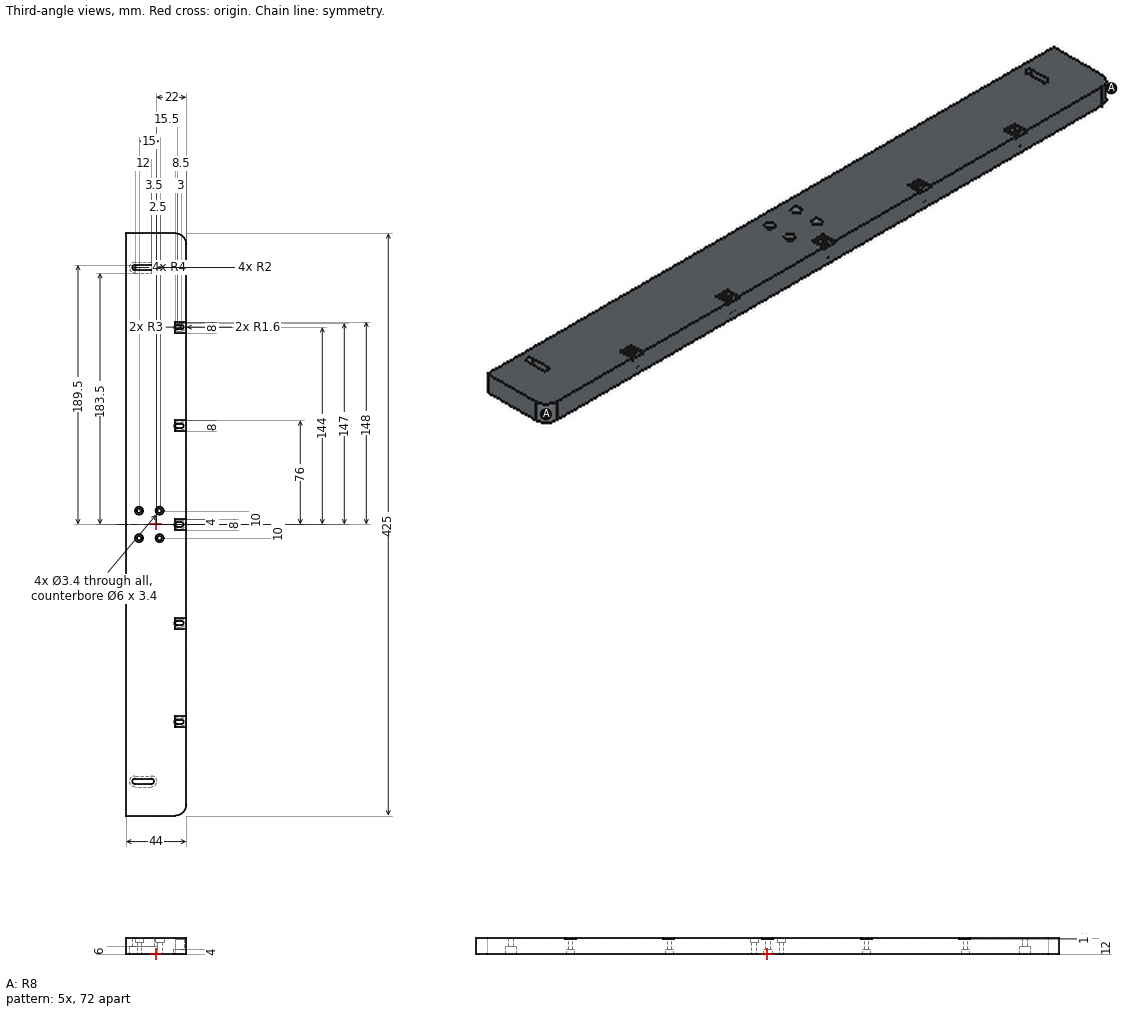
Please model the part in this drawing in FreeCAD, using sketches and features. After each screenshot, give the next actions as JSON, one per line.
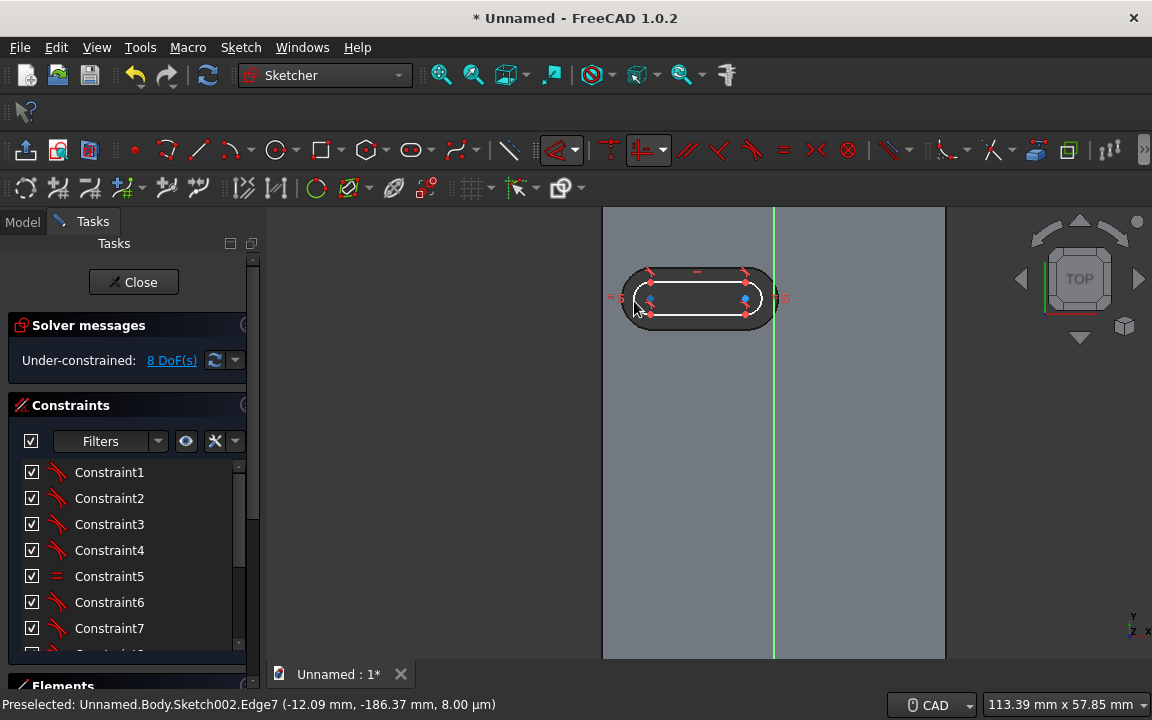
{"action": "left_click", "coordinate": [634, 299]}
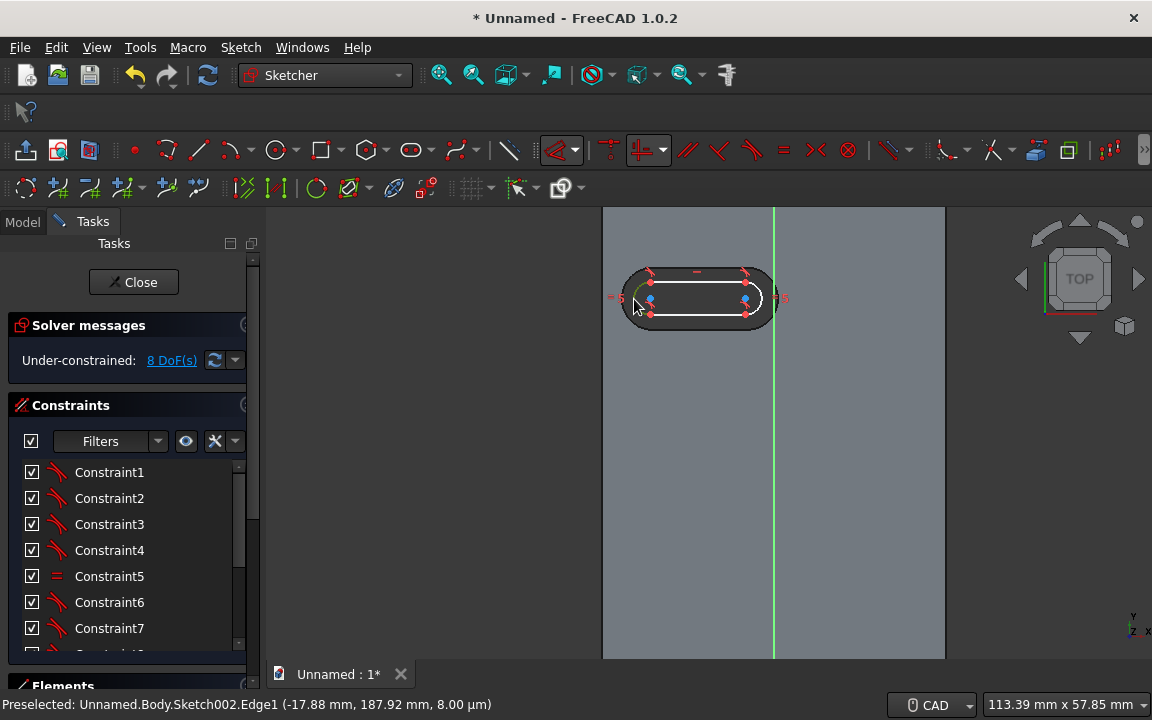
{"action": "scroll", "coordinate": [634, 300], "scroll_direction": "down", "scroll_amount": 12}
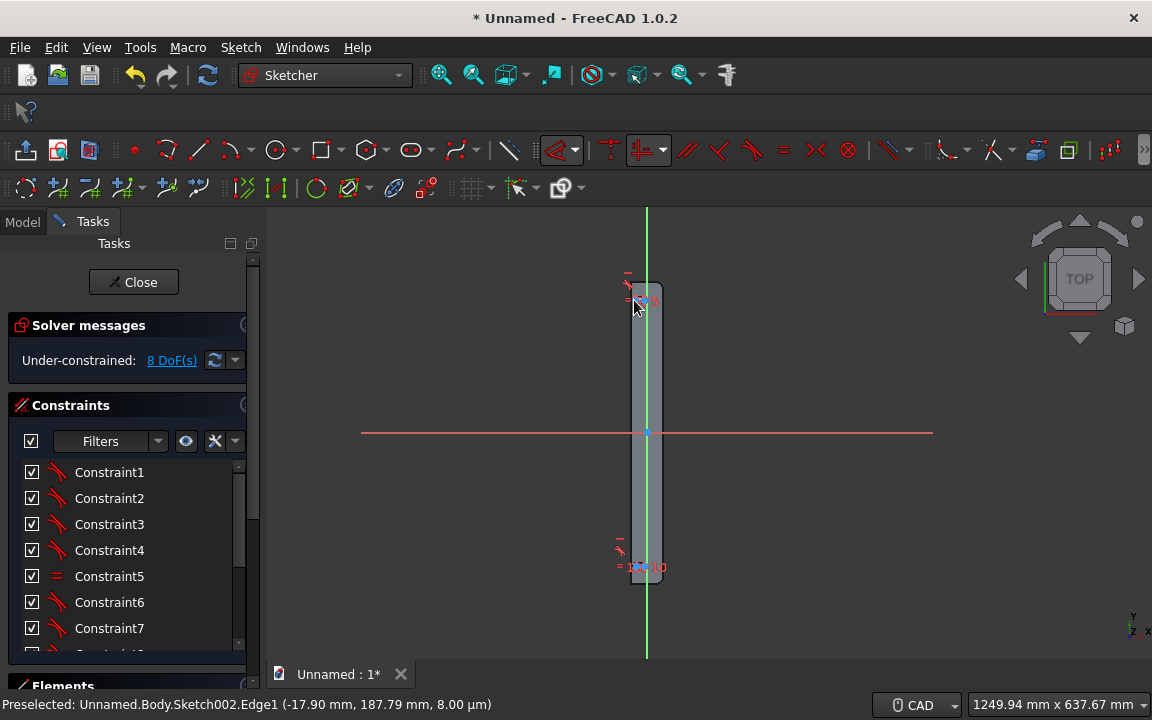
{"action": "scroll", "coordinate": [635, 566], "scroll_direction": "up", "scroll_amount": 14}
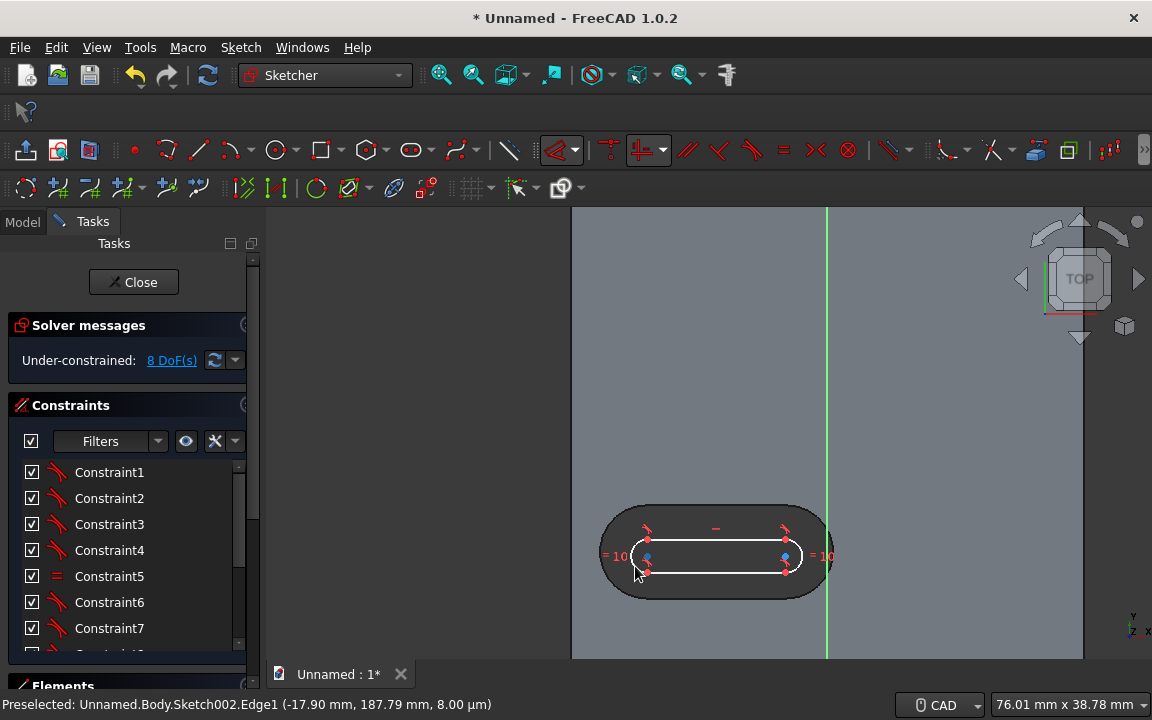
{"action": "left_click", "coordinate": [634, 546]}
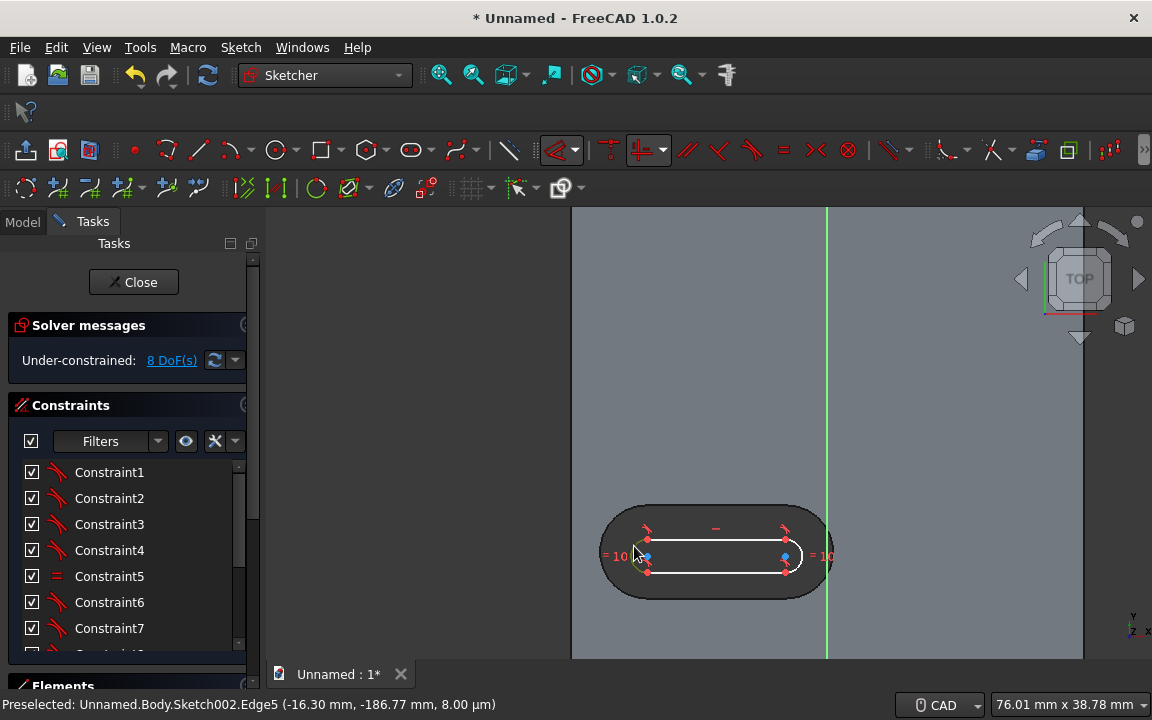
{"action": "key", "text": "e"}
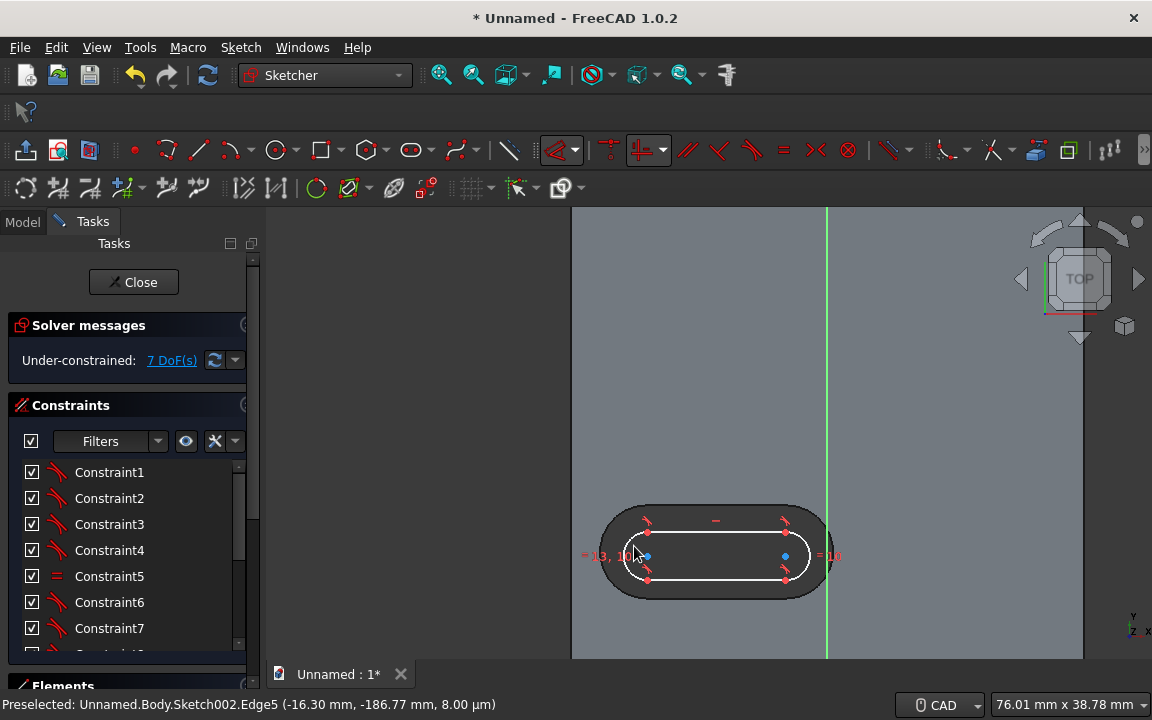
{"action": "scroll", "coordinate": [635, 567], "scroll_direction": "down", "scroll_amount": 14}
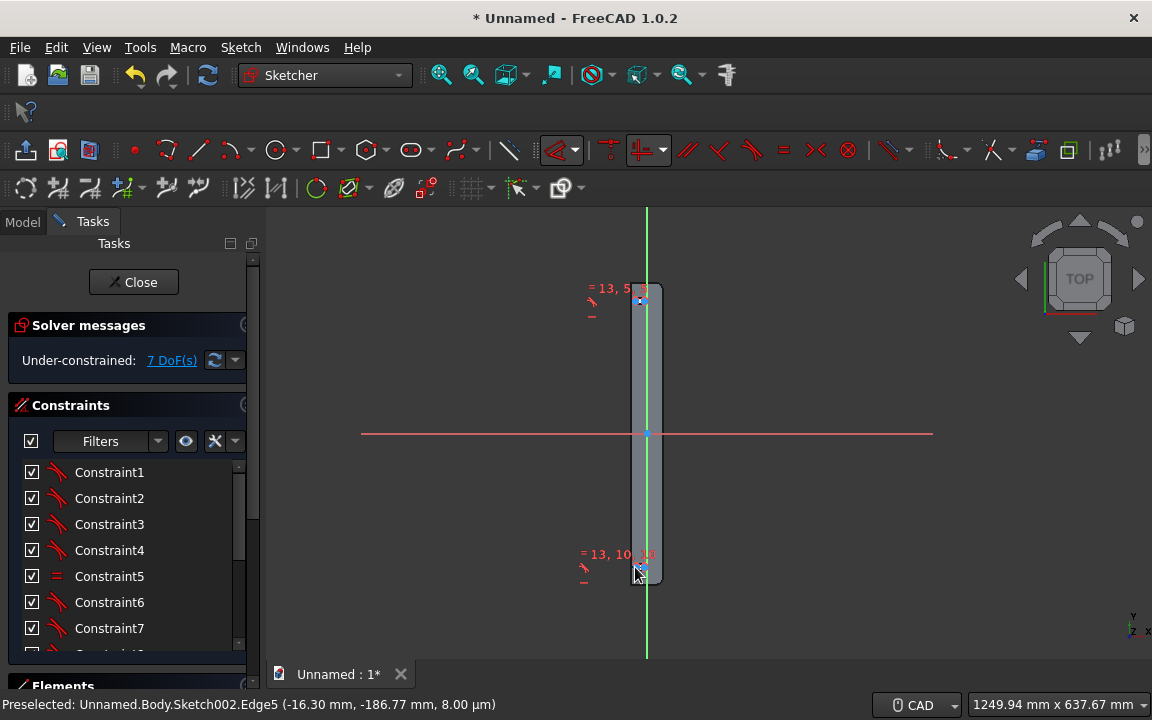
{"action": "scroll", "coordinate": [636, 301], "scroll_direction": "up", "scroll_amount": 11}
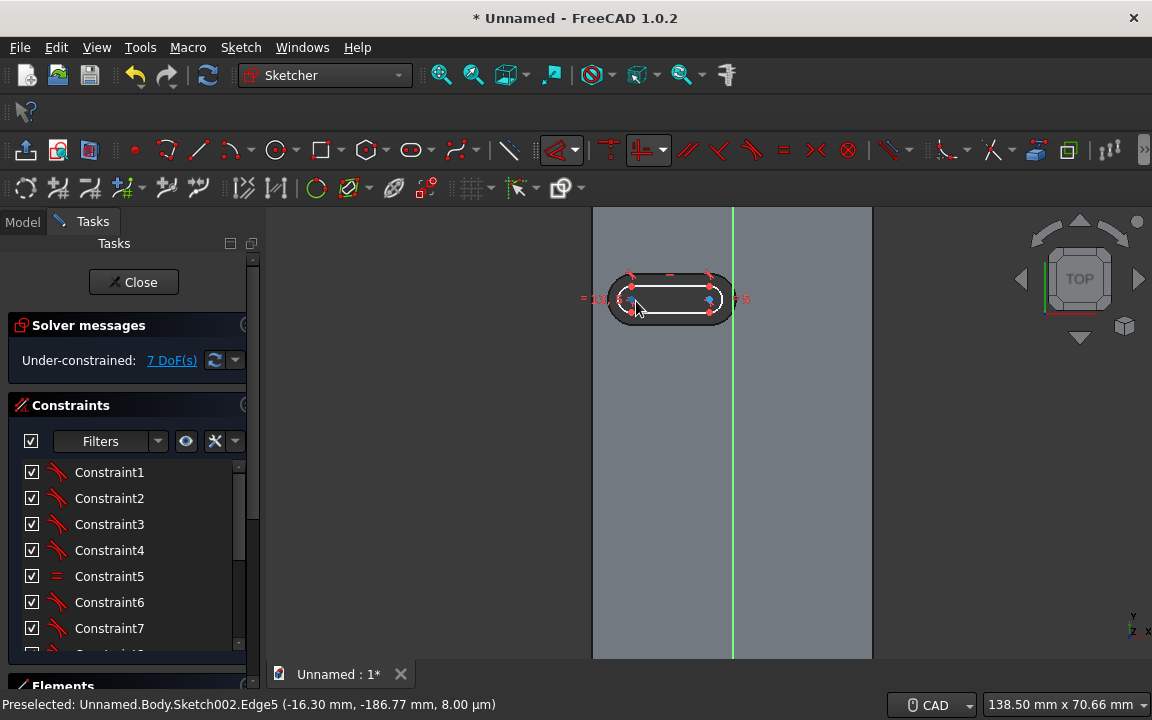
{"action": "left_click", "coordinate": [631, 299]}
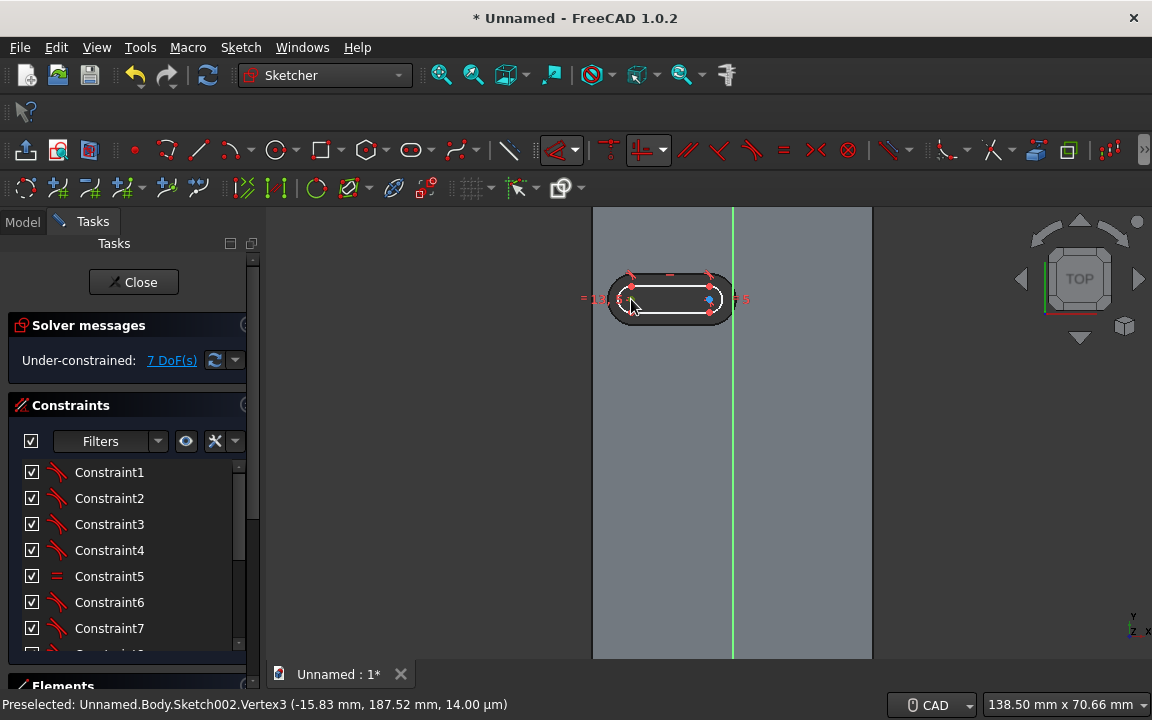
{"action": "scroll", "coordinate": [636, 300], "scroll_direction": "down", "scroll_amount": 11}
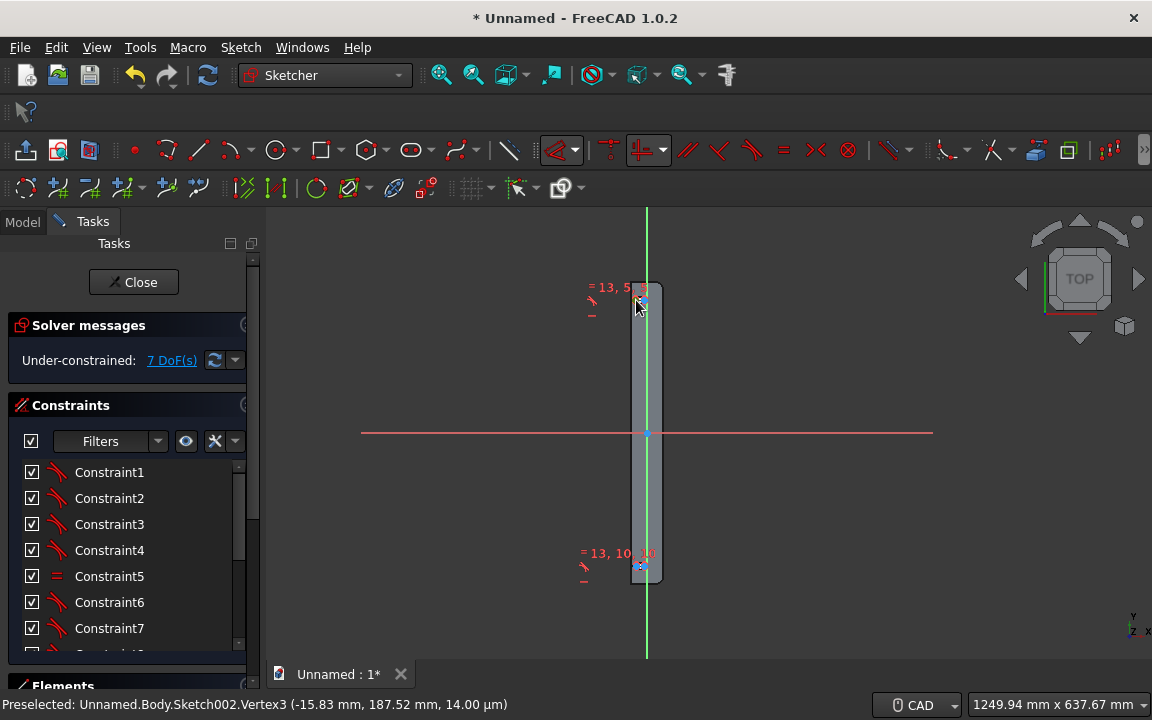
{"action": "scroll", "coordinate": [636, 566], "scroll_direction": "up", "scroll_amount": 11}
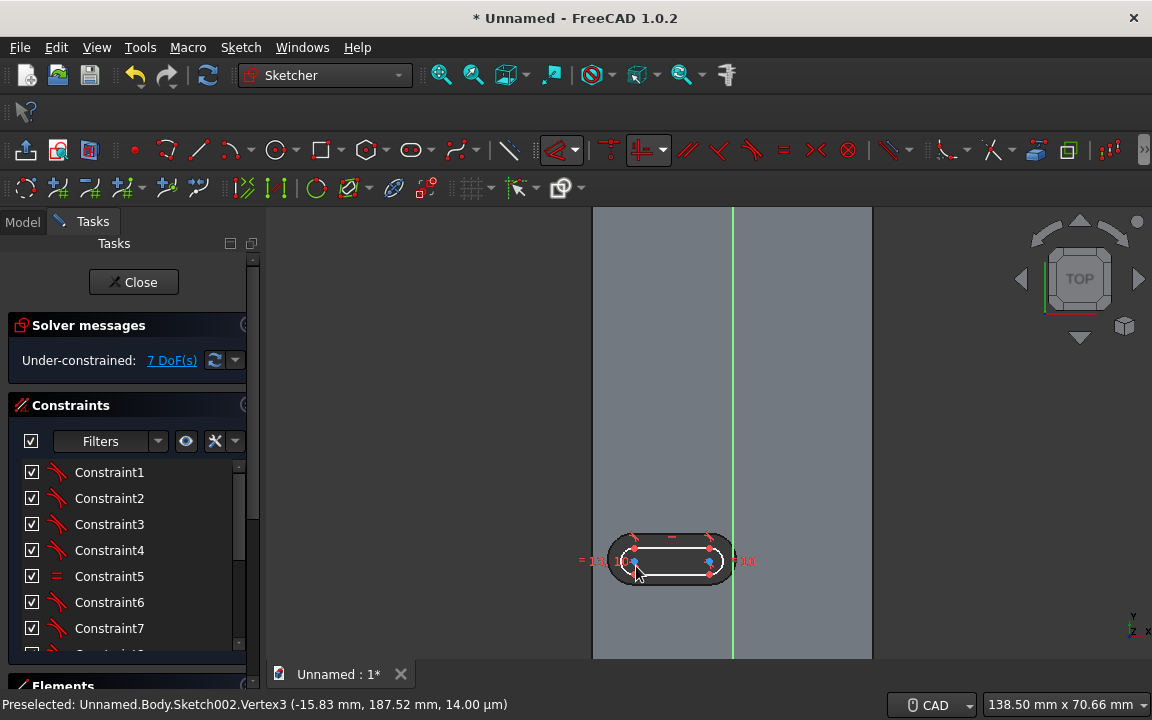
{"action": "left_click", "coordinate": [634, 561]}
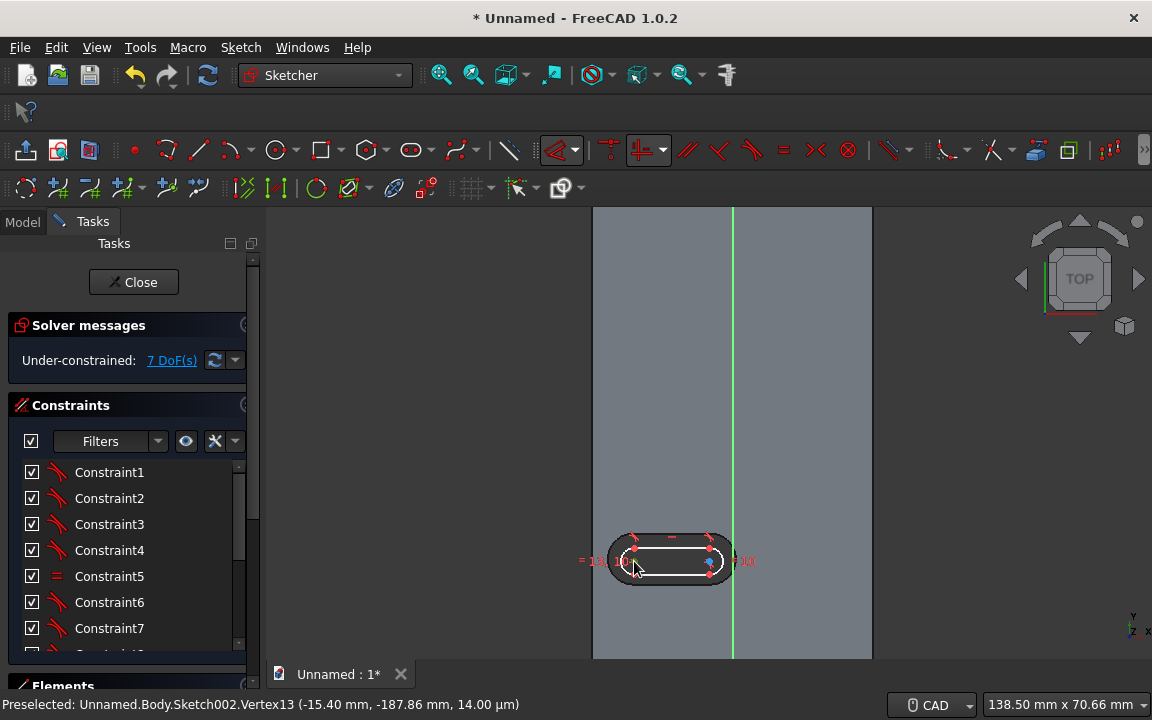
{"action": "scroll", "coordinate": [636, 567], "scroll_direction": "down", "scroll_amount": 11}